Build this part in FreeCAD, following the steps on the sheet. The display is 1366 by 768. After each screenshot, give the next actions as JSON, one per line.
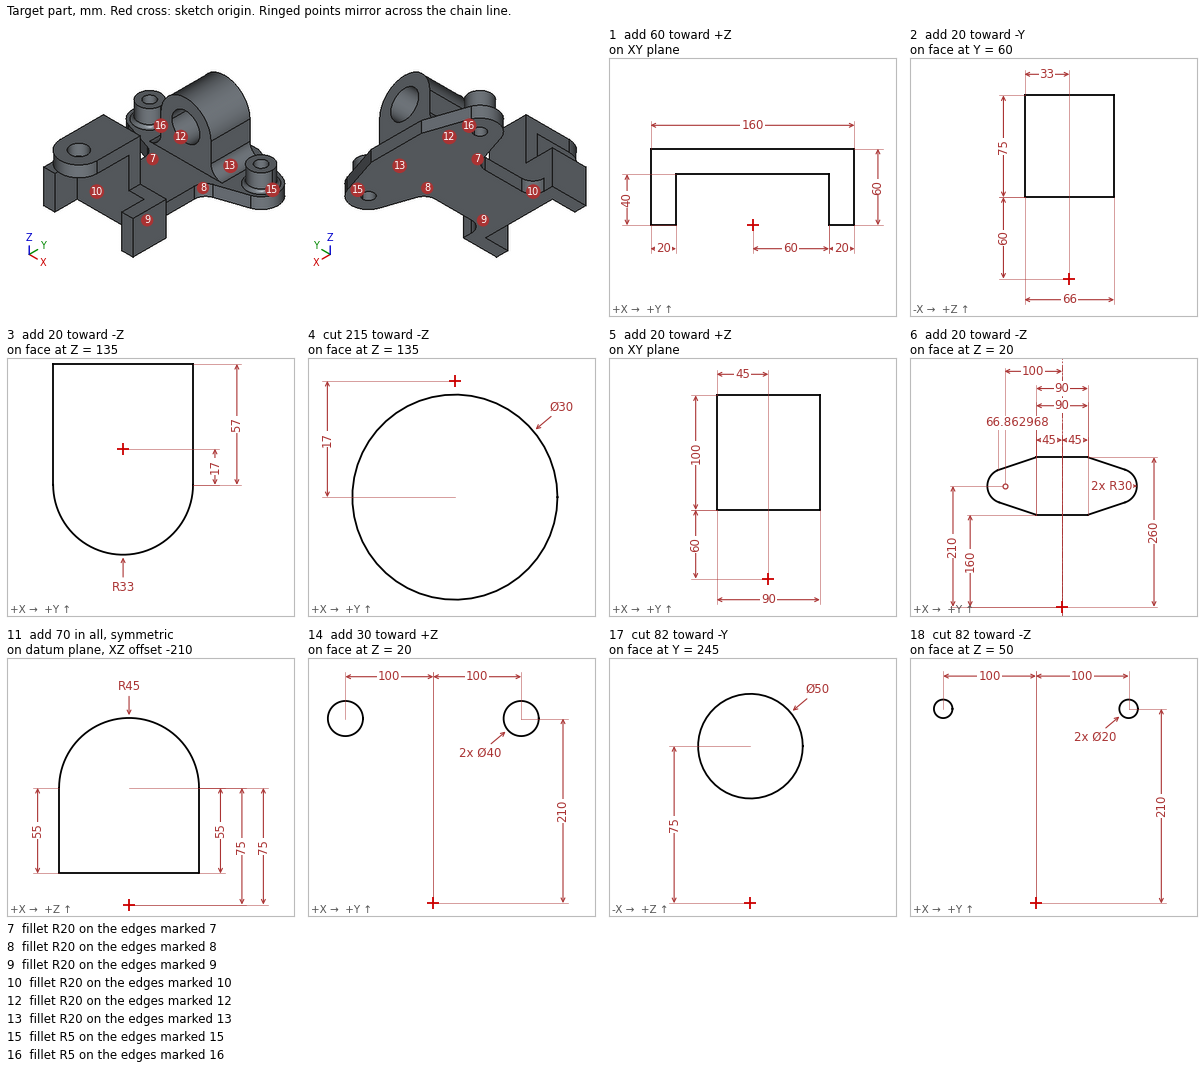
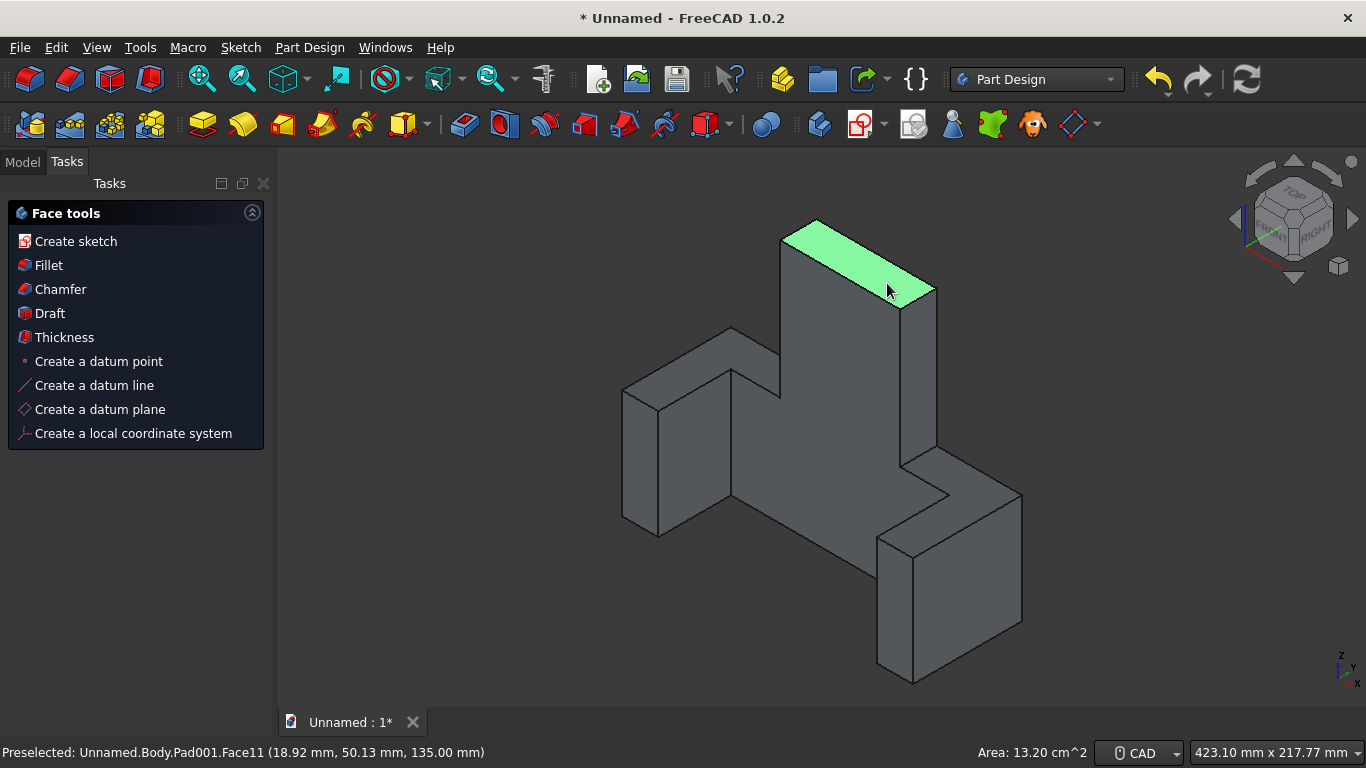
{"action": "left_click", "coordinate": [860, 124]}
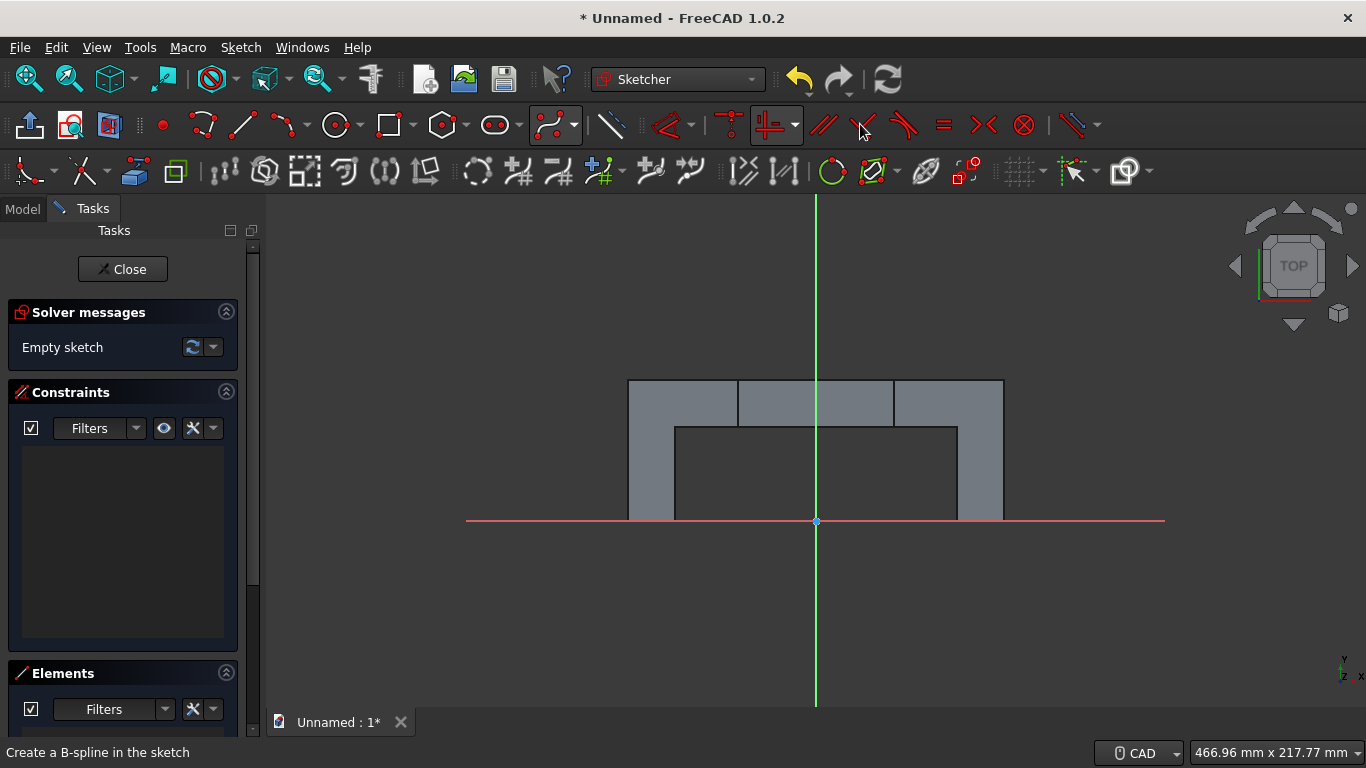
{"action": "scroll", "coordinate": [955, 679], "scroll_direction": "up", "scroll_amount": 2}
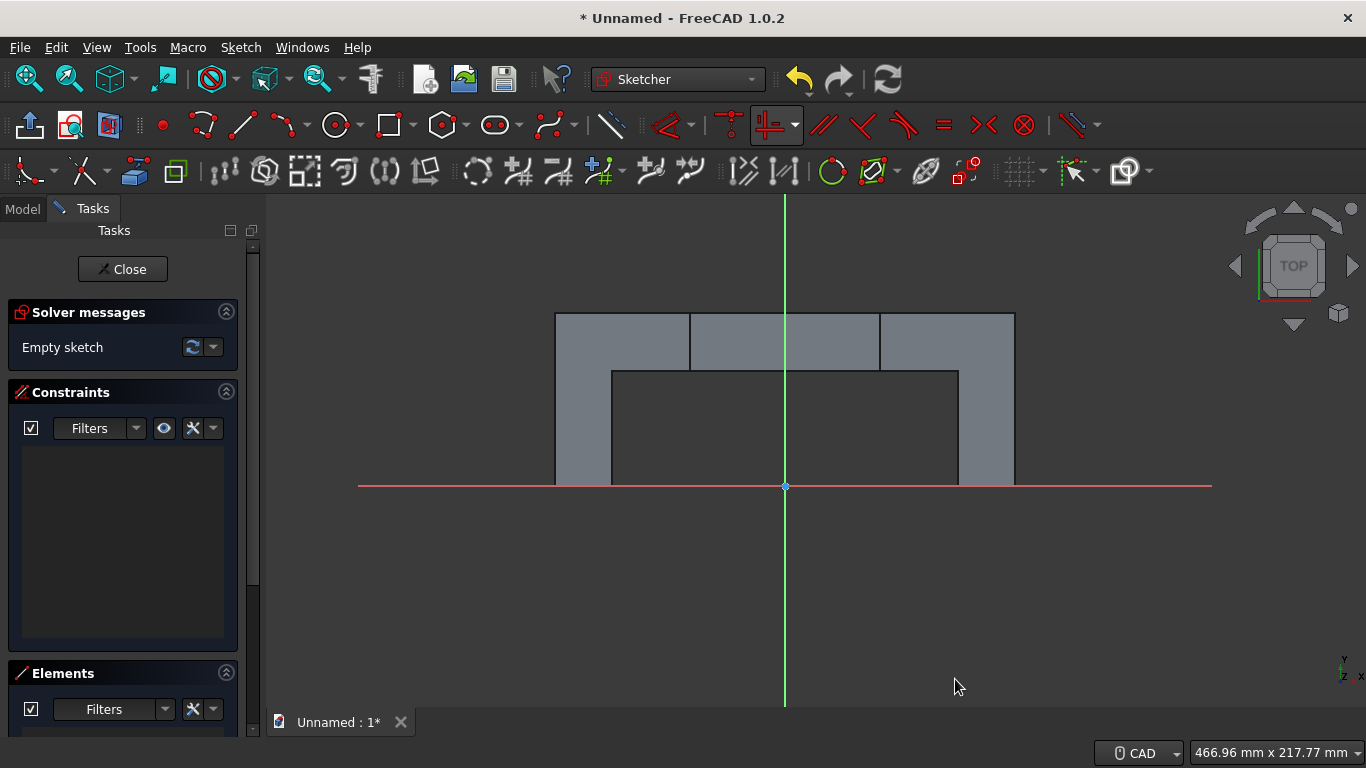
{"action": "left_click", "coordinate": [204, 126]}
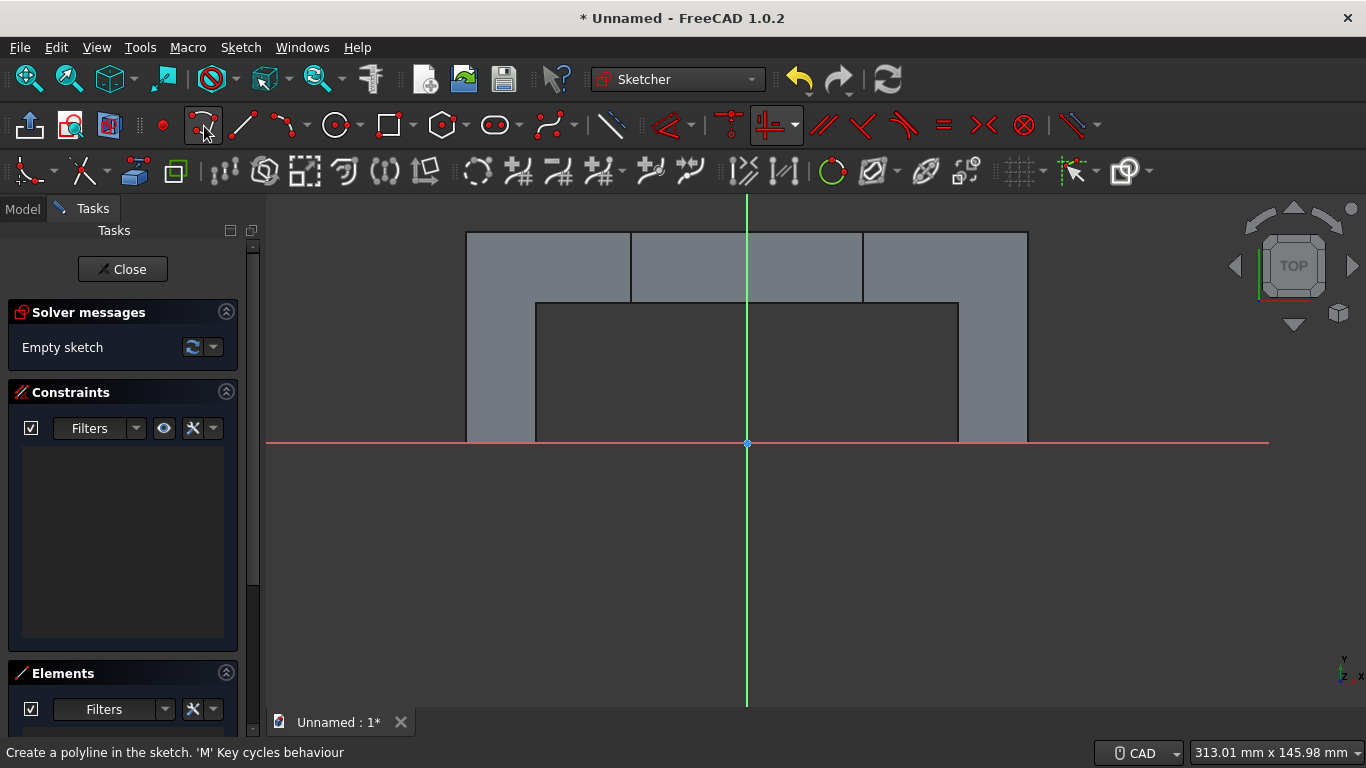
{"action": "left_click", "coordinate": [863, 503]}
{"action": "left_click", "coordinate": [863, 303]}
{"action": "left_click", "coordinate": [631, 303]}
{"action": "left_click", "coordinate": [631, 503]}
{"action": "right_click", "coordinate": [631, 503]}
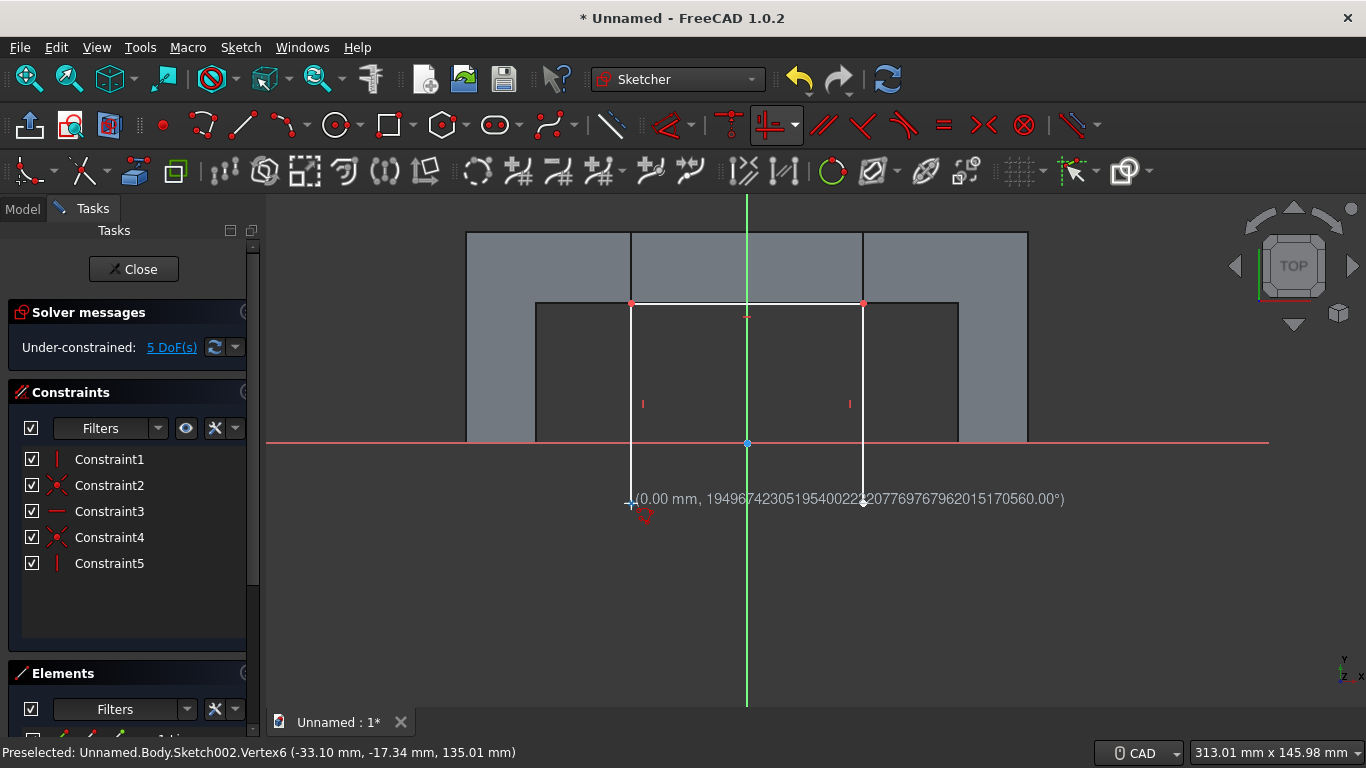
{"action": "key", "text": "g 3 a"}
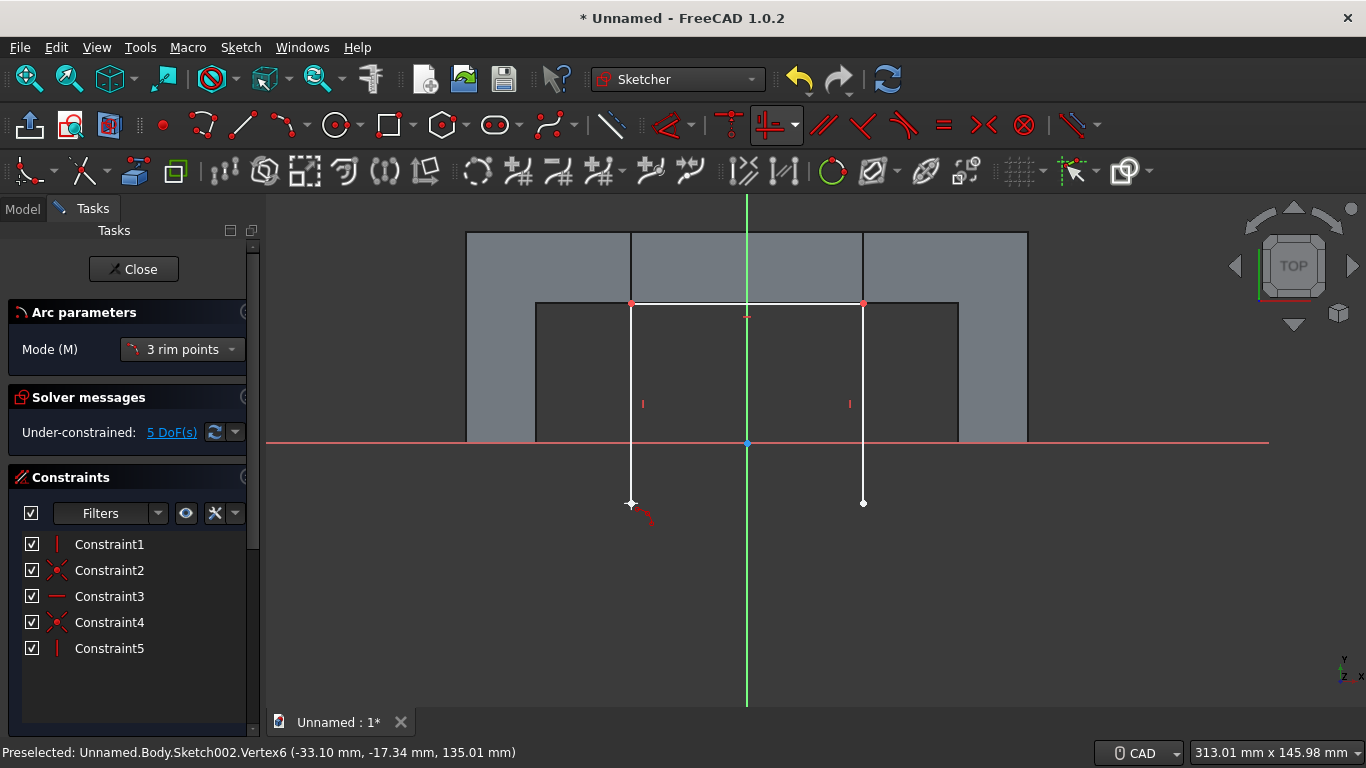
{"action": "left_click", "coordinate": [631, 504]}
{"action": "left_click", "coordinate": [863, 504]}
{"action": "left_click", "coordinate": [711, 613]}
{"action": "key", "text": "Escape"}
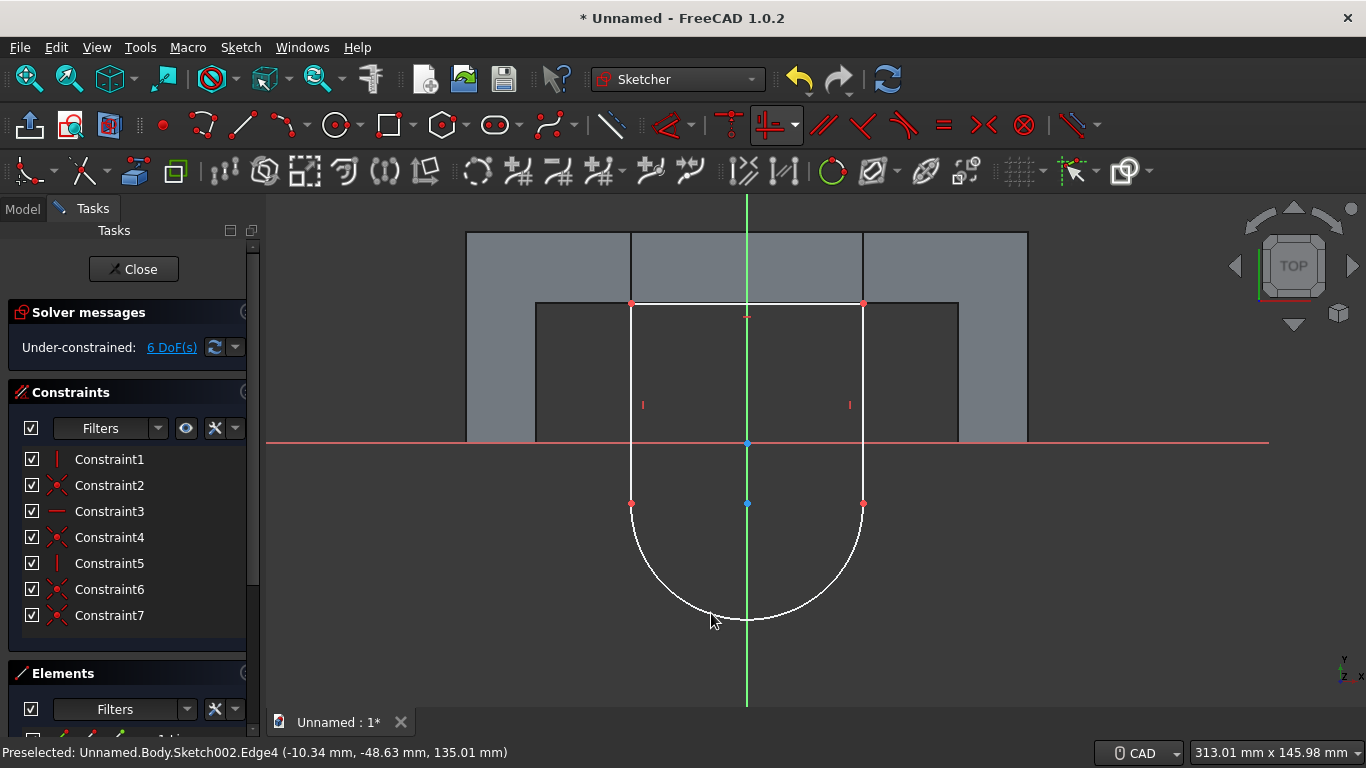
{"action": "left_click", "coordinate": [863, 444]}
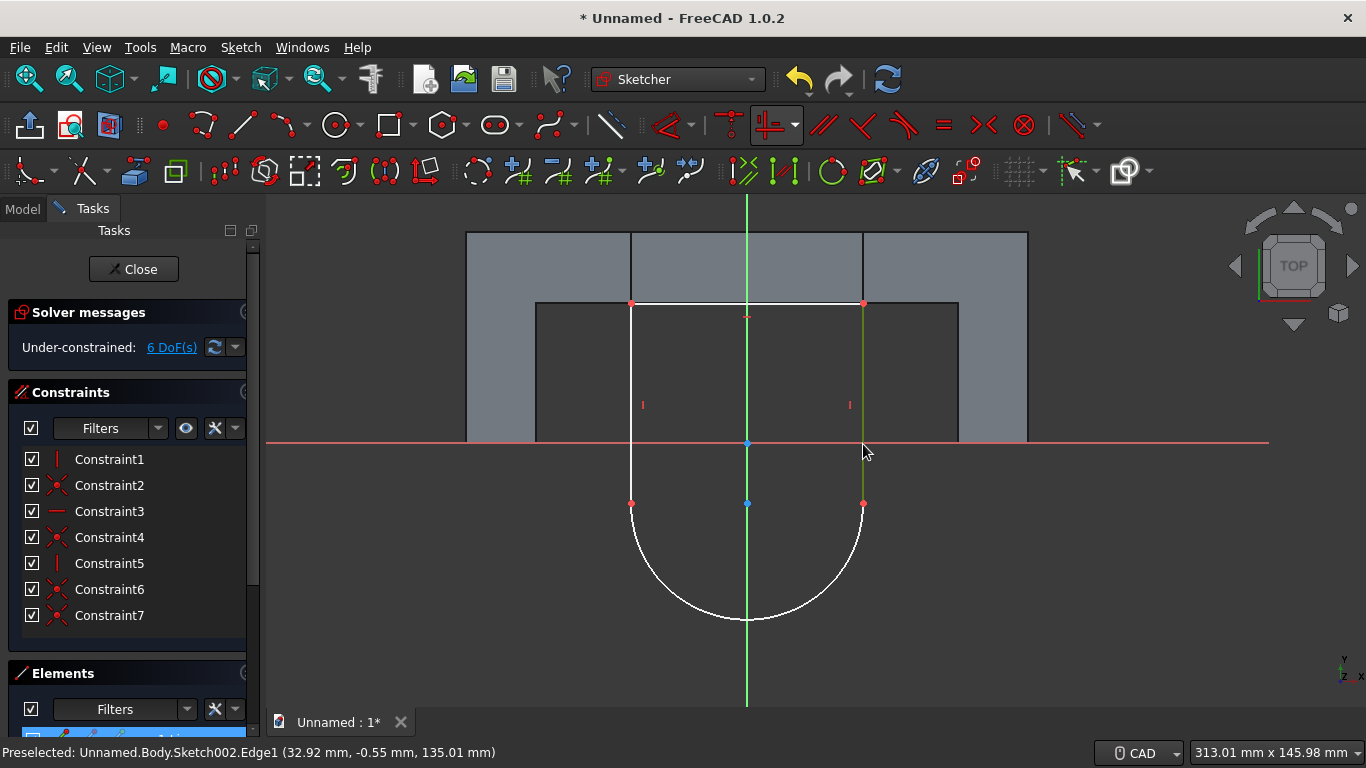
{"action": "left_click", "coordinate": [679, 598]}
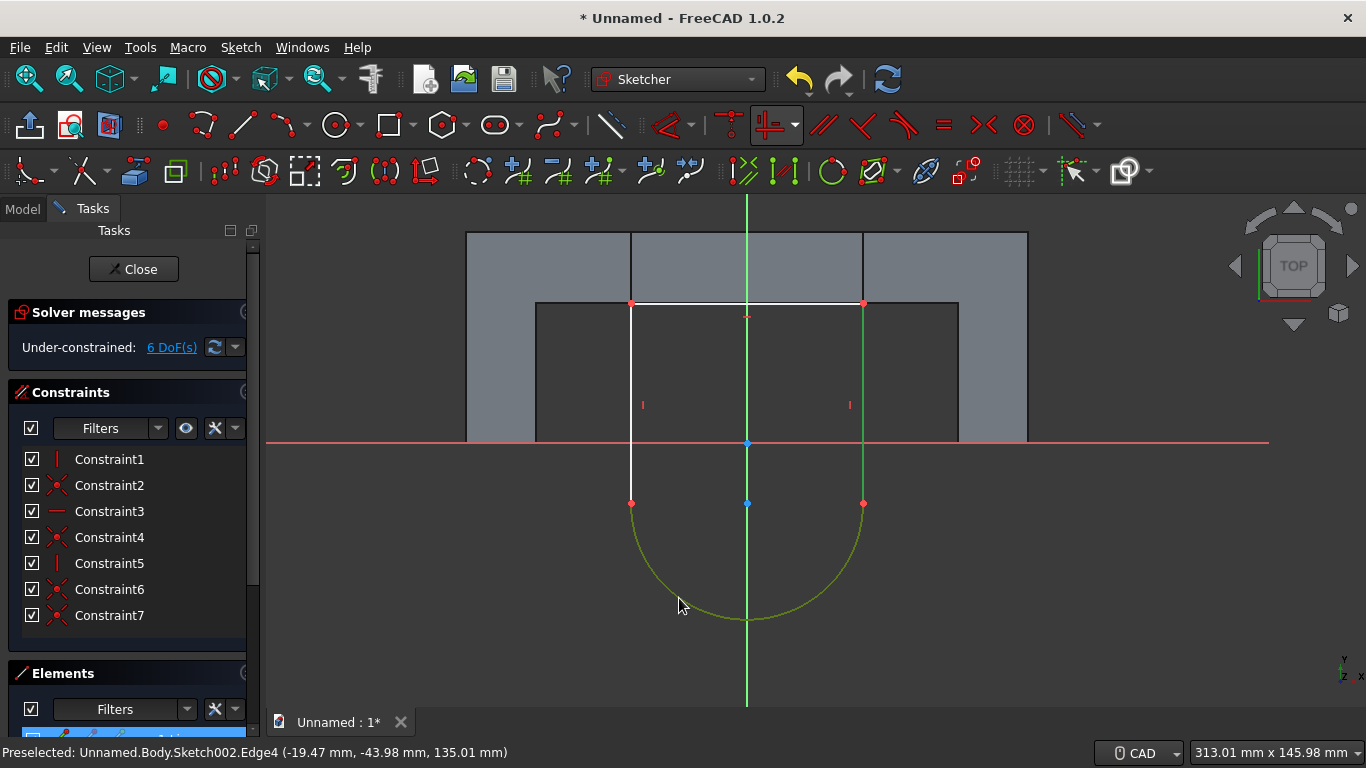
{"action": "key", "text": "t"}